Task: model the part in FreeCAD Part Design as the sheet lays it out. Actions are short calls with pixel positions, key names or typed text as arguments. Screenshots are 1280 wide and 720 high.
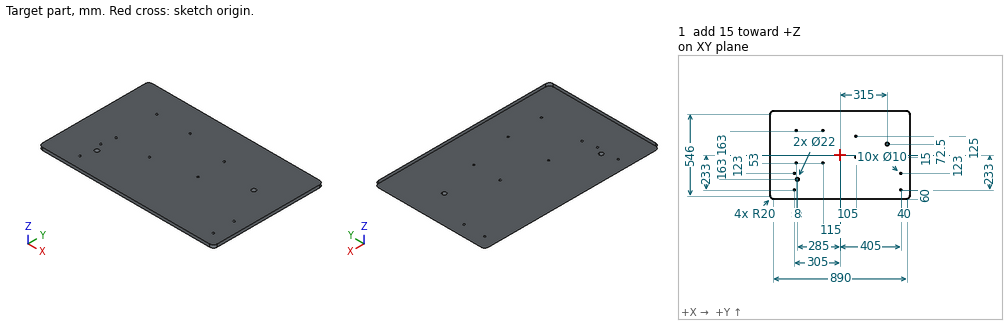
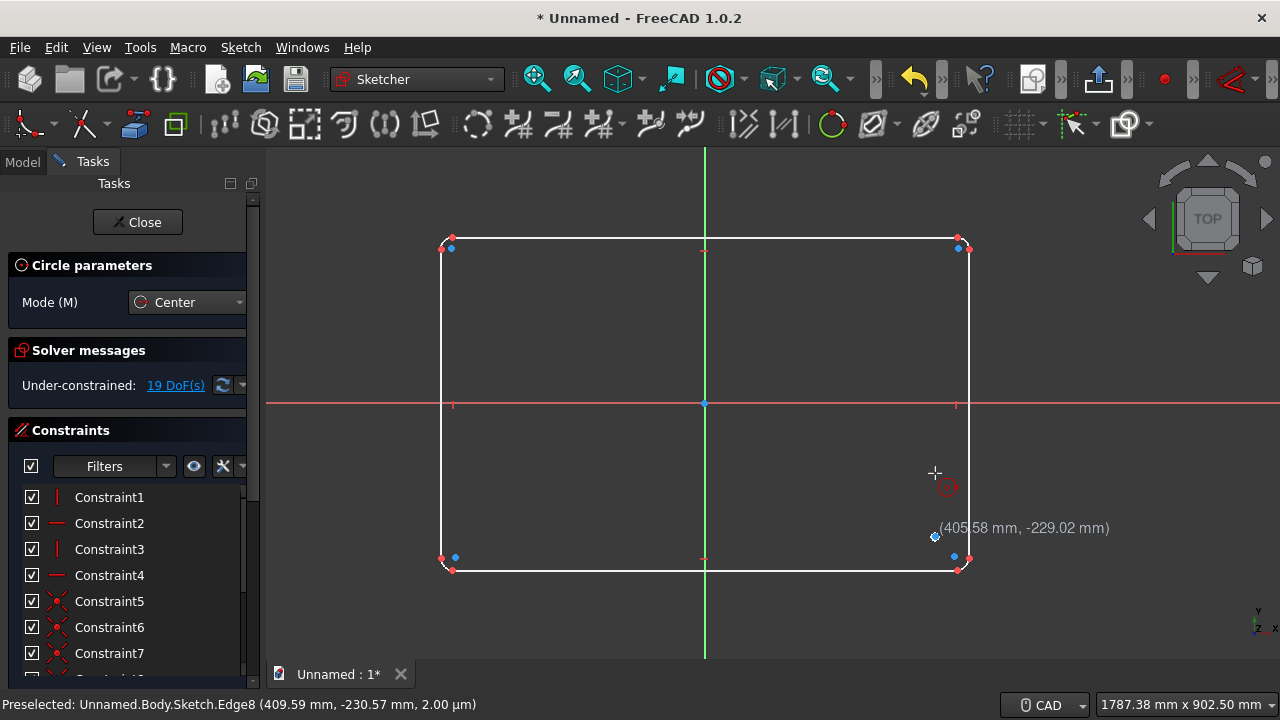
click(935, 473)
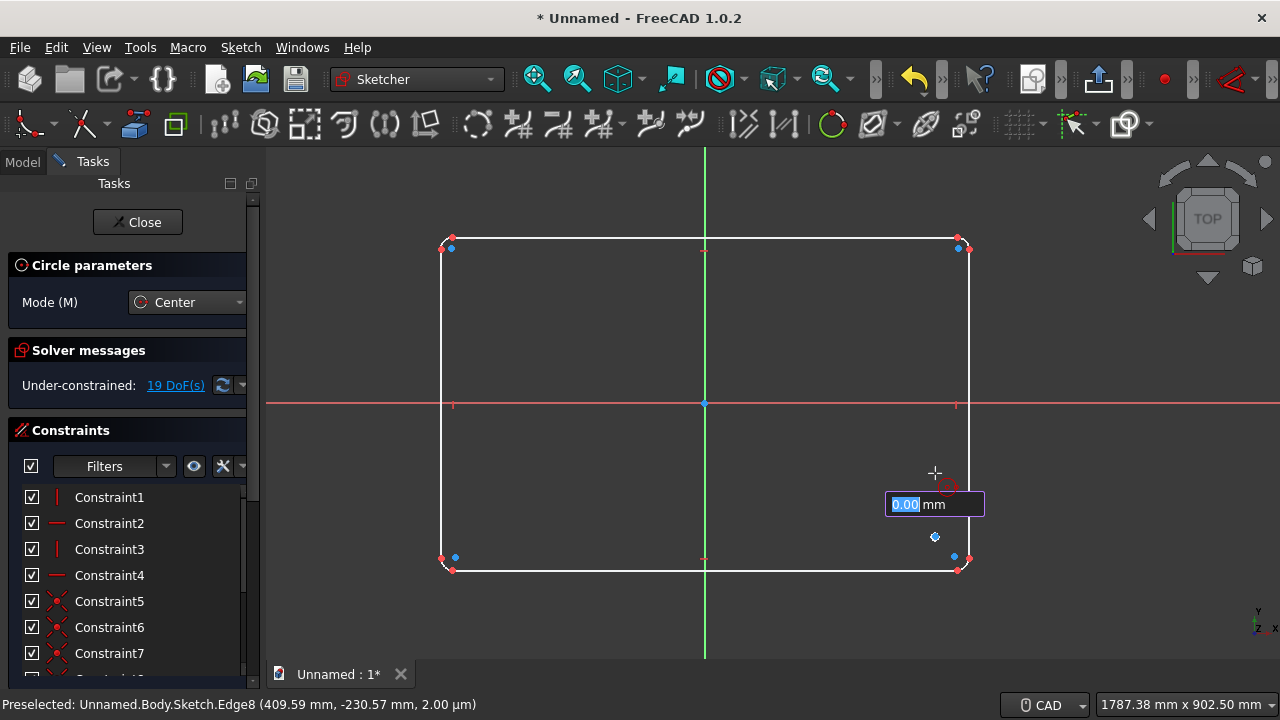
scroll(937, 471, up, 9)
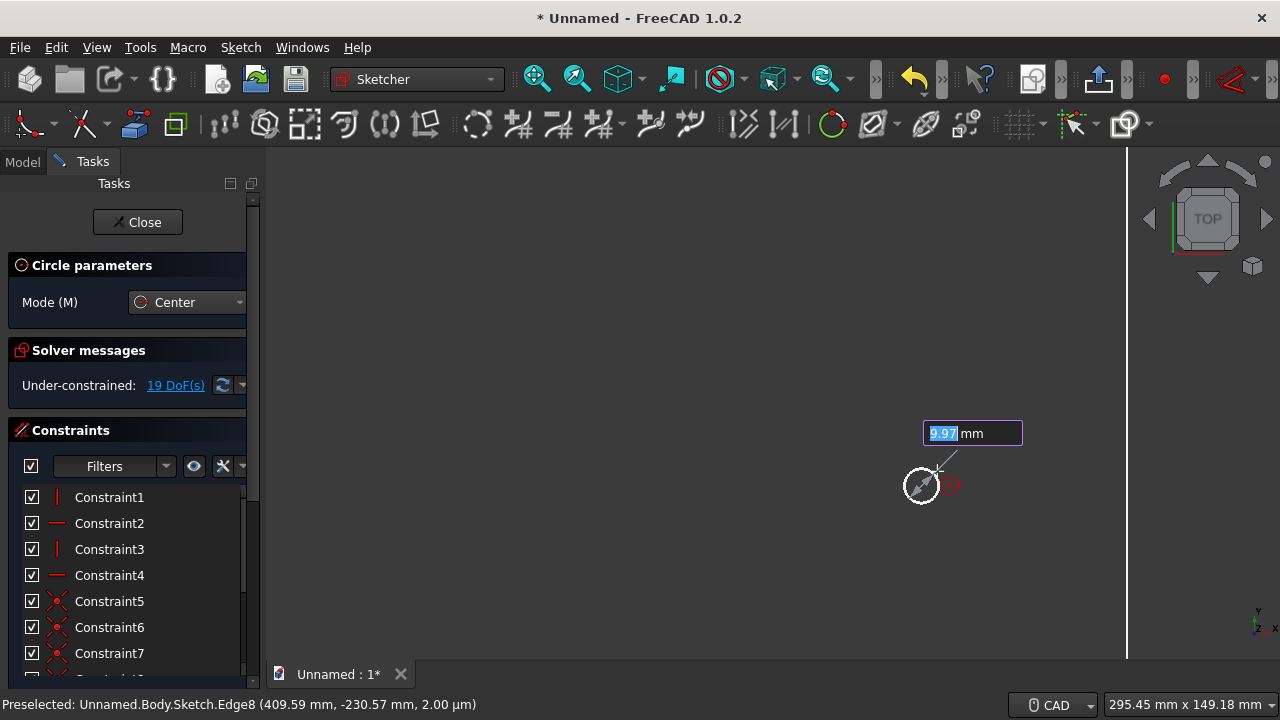
click(932, 469)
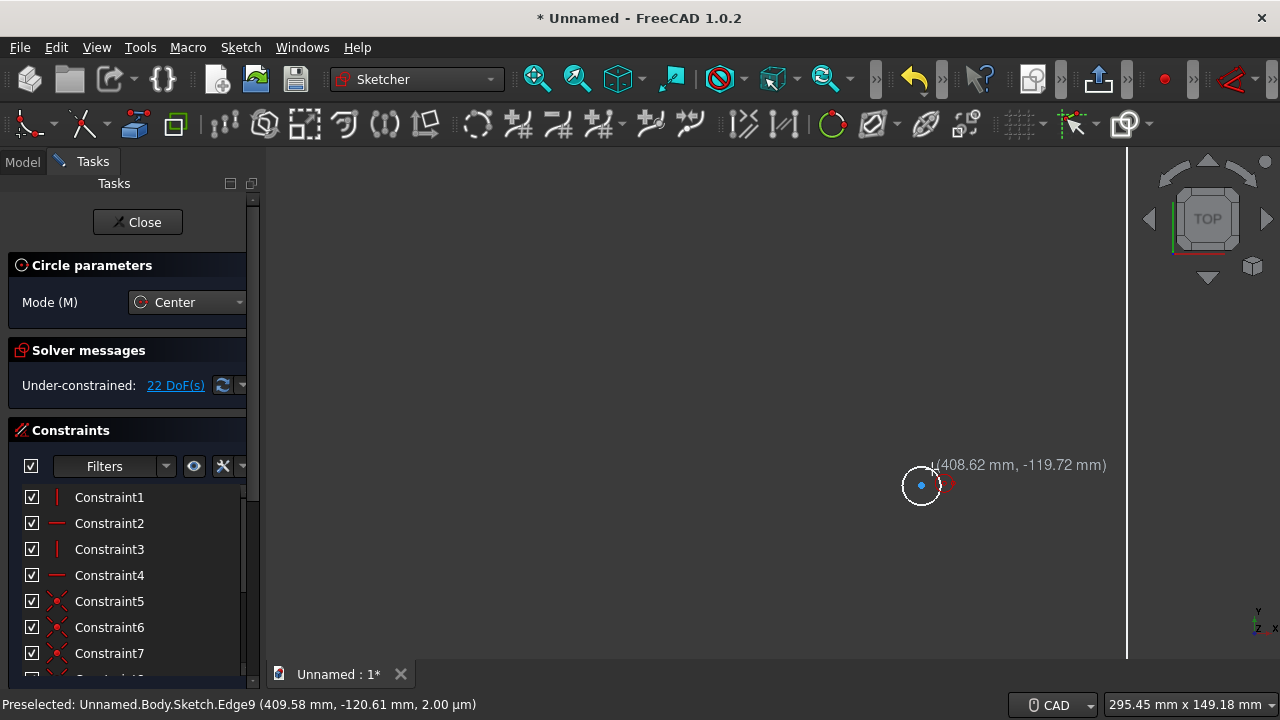
scroll(937, 471, down, 9)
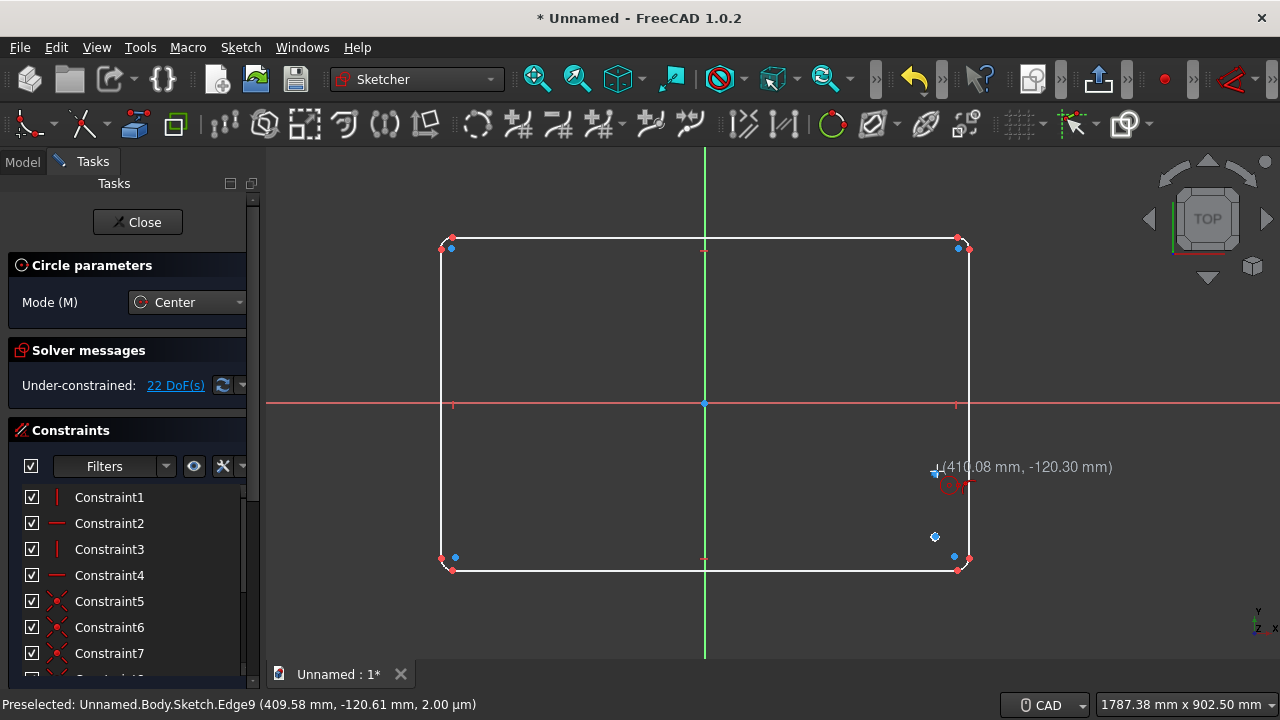
scroll(532, 536, up, 11)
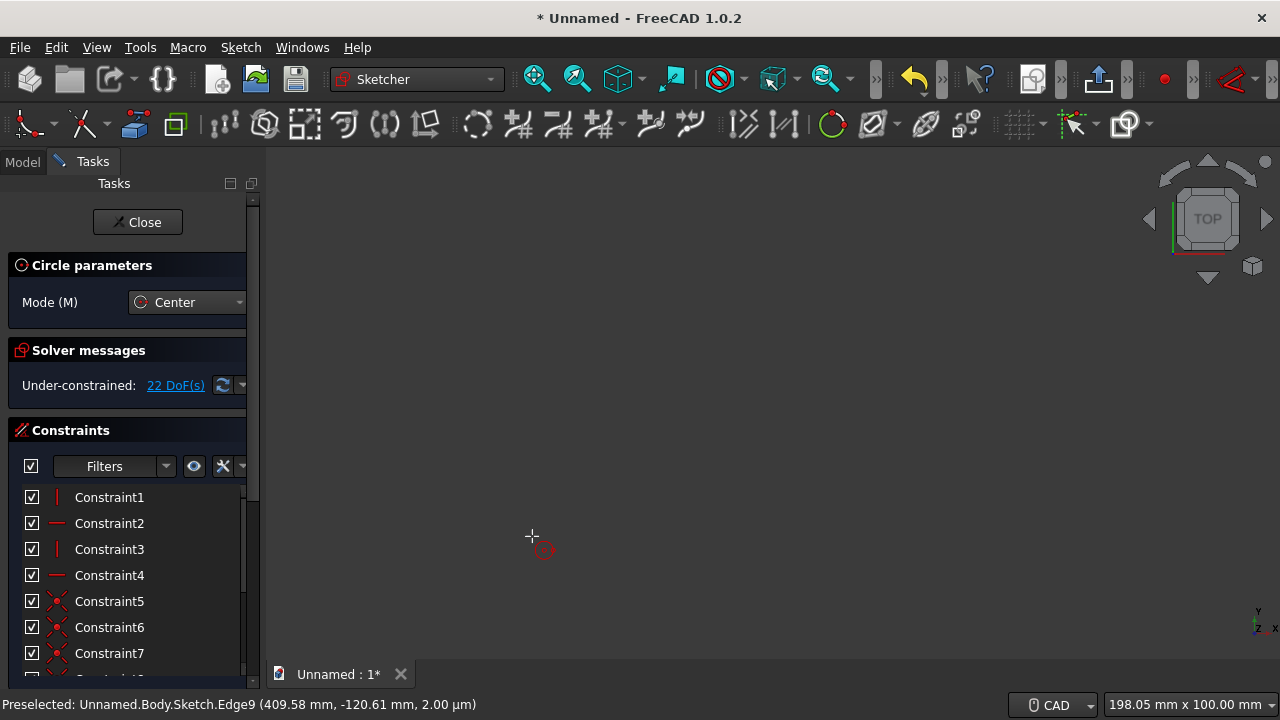
scroll(532, 536, down, 11)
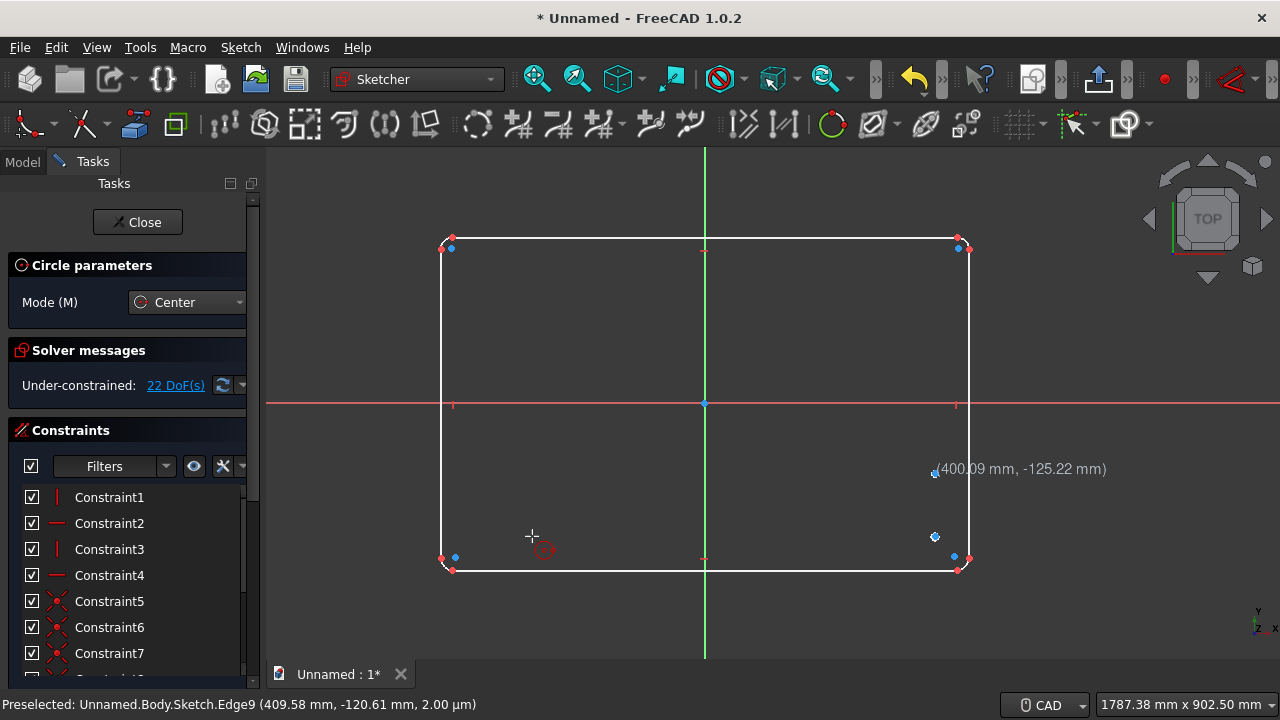
click(532, 536)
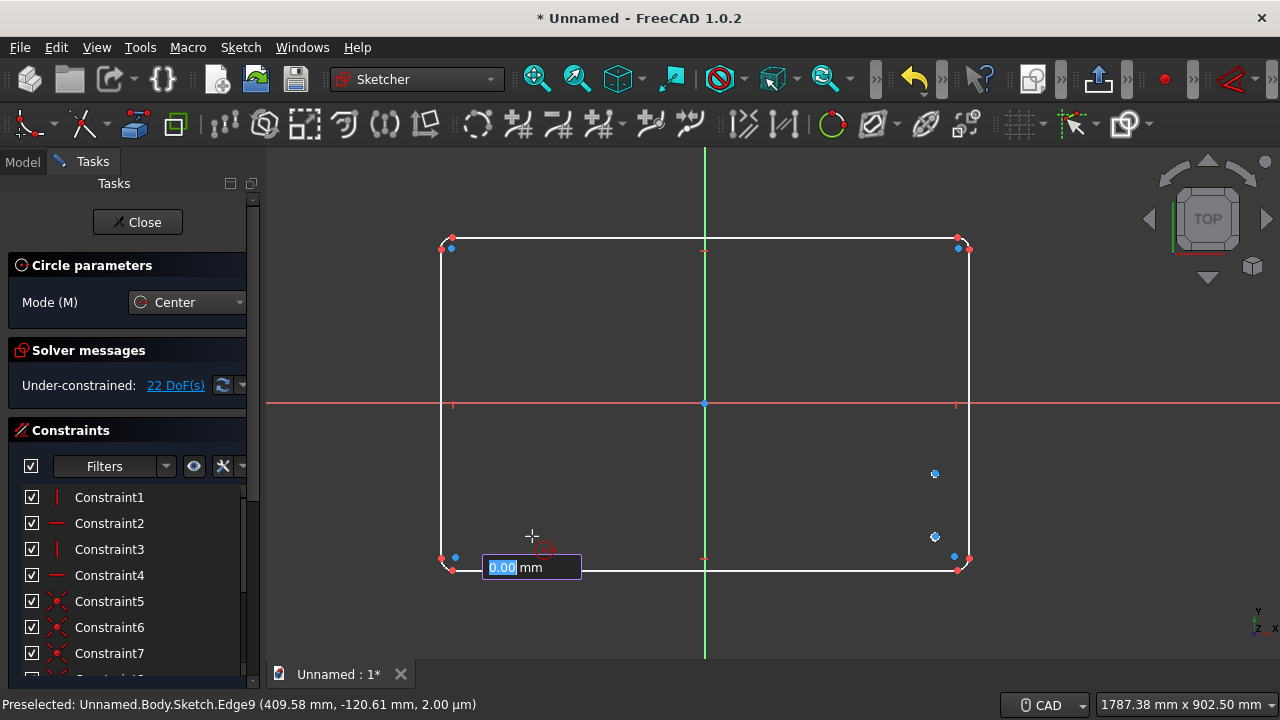
scroll(534, 534, up, 9)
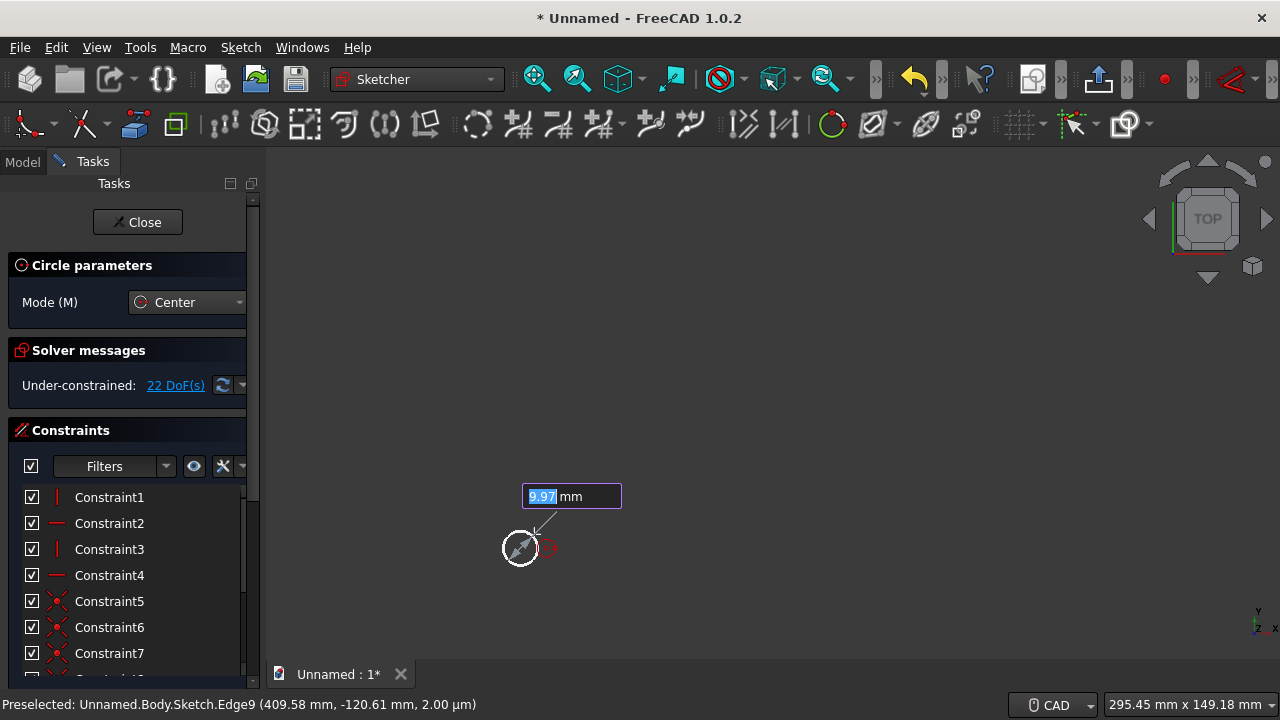
click(532, 528)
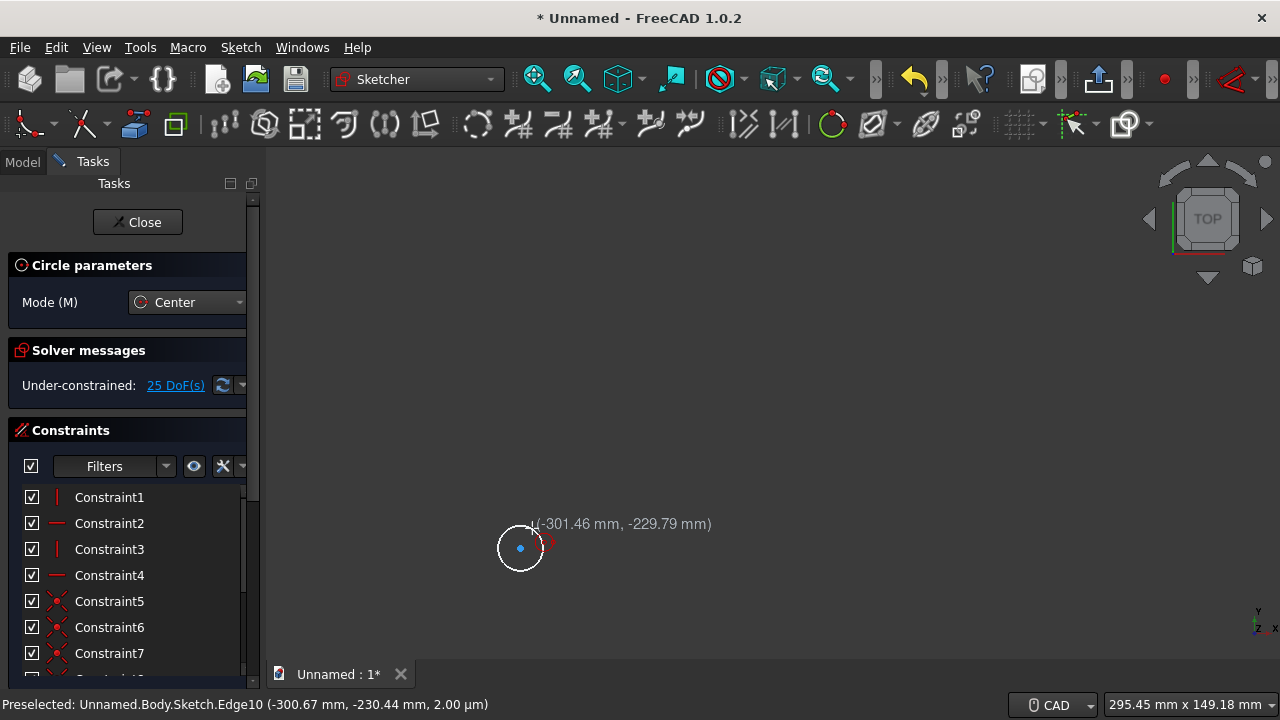
scroll(534, 534, down, 9)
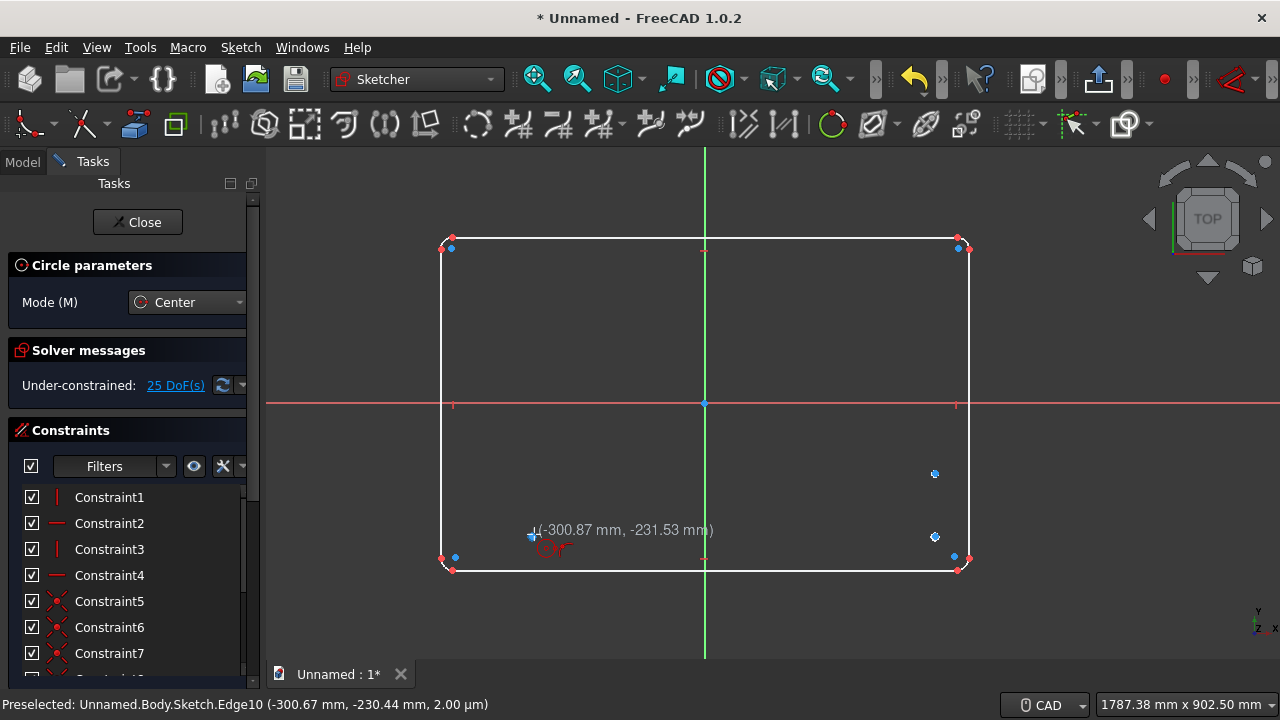
click(543, 496)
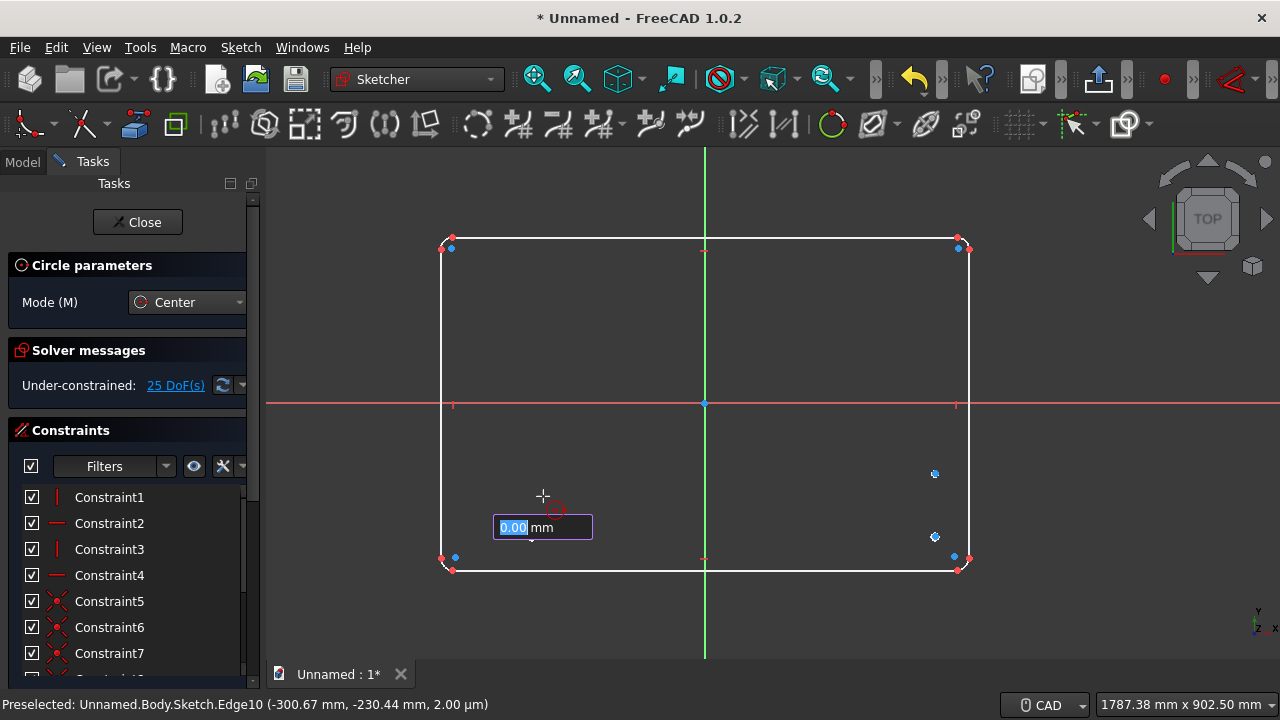
scroll(548, 492, up, 5)